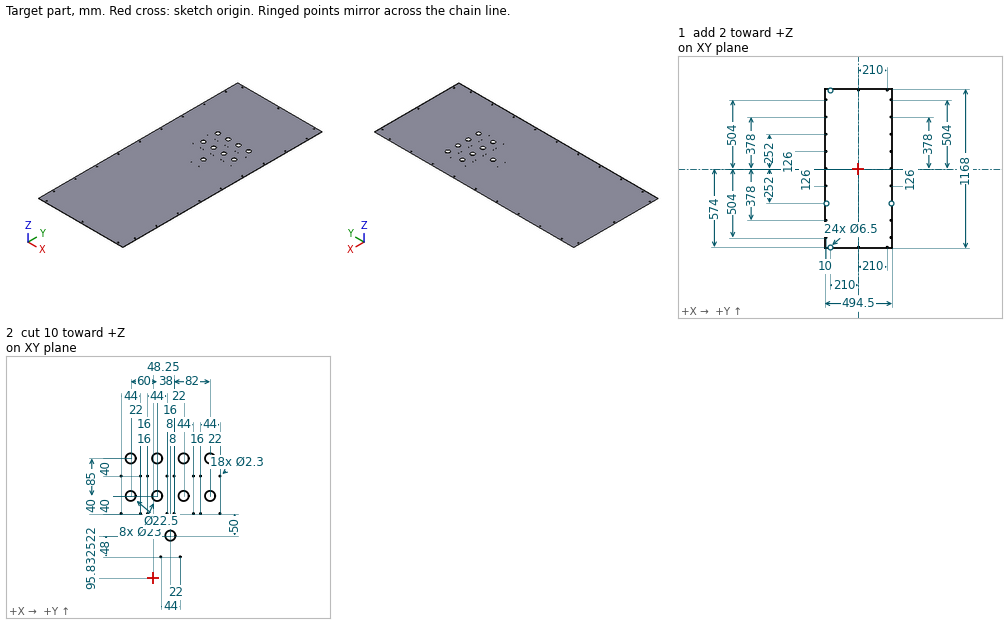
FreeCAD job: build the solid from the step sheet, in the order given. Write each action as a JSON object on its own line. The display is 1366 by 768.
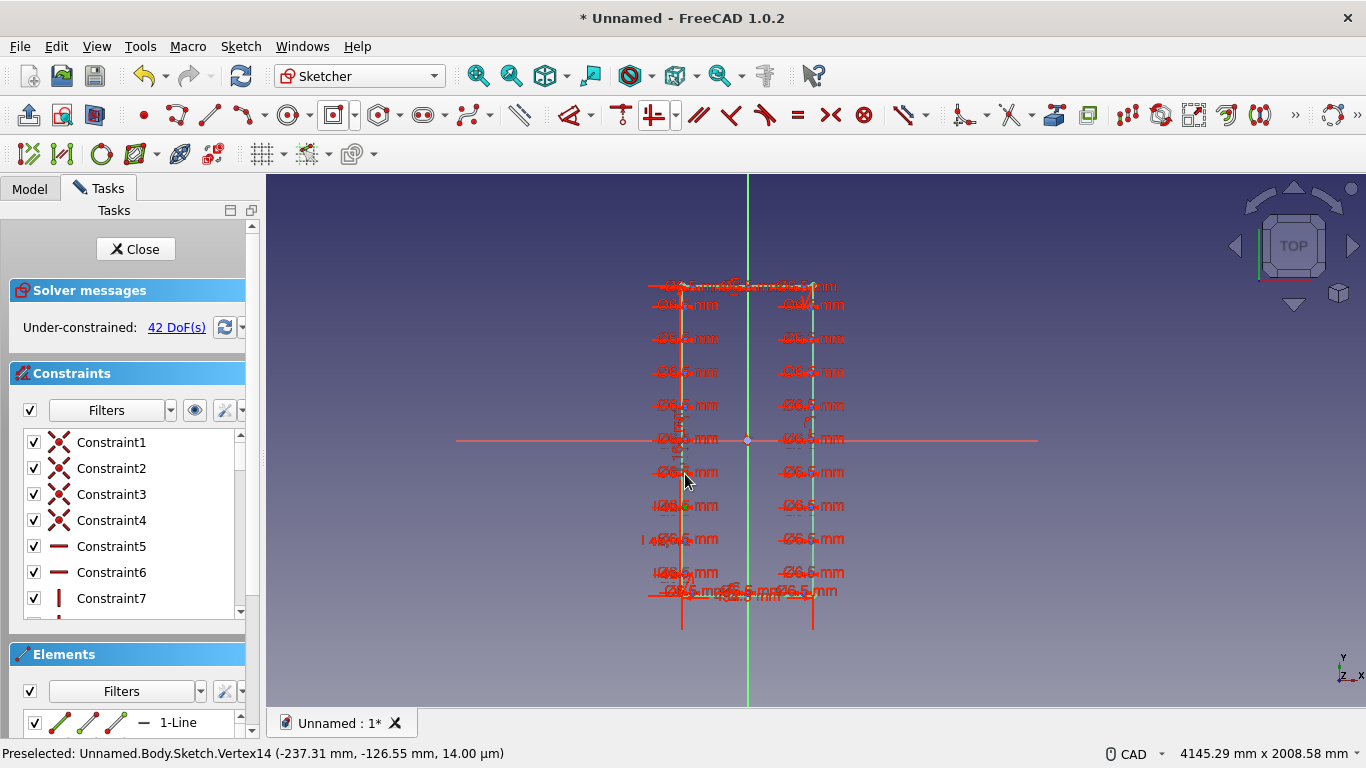
{"action": "key", "text": "v"}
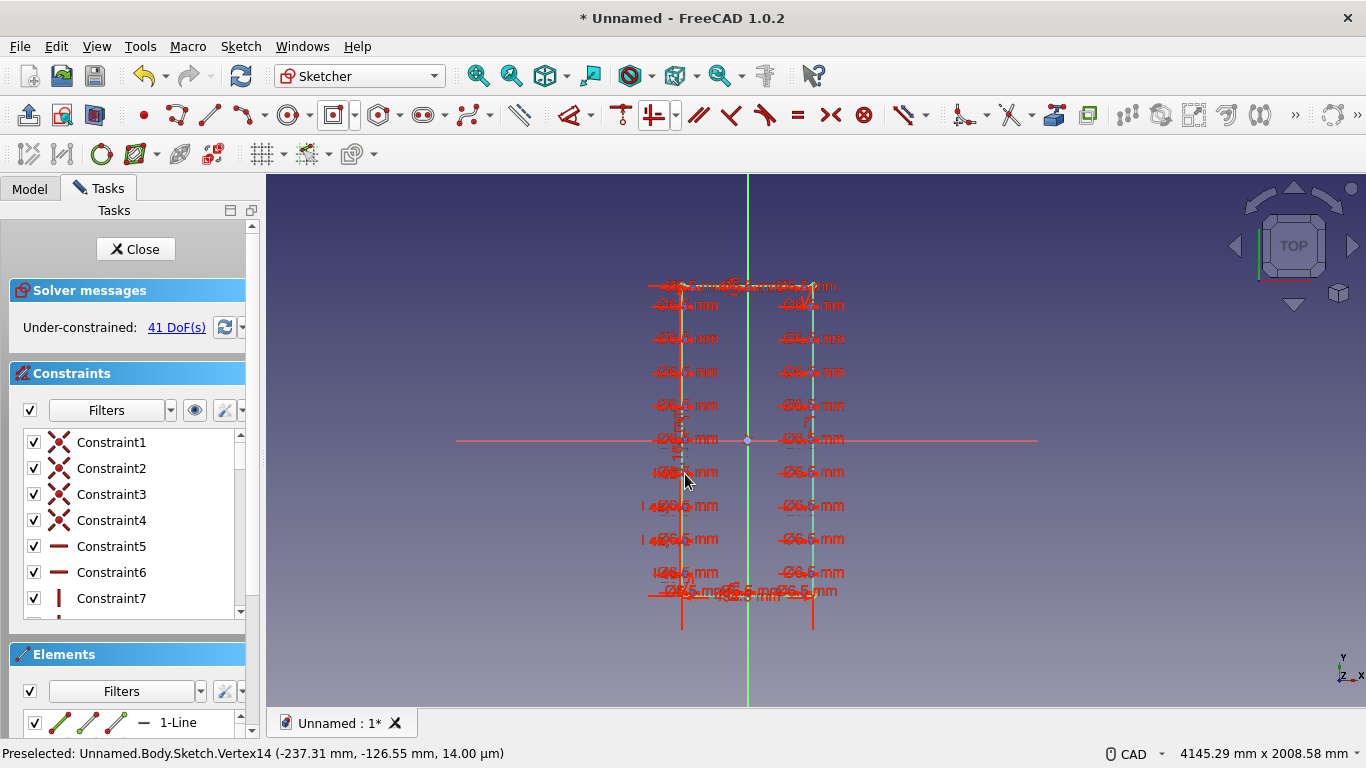
{"action": "left_click", "coordinate": [692, 593]}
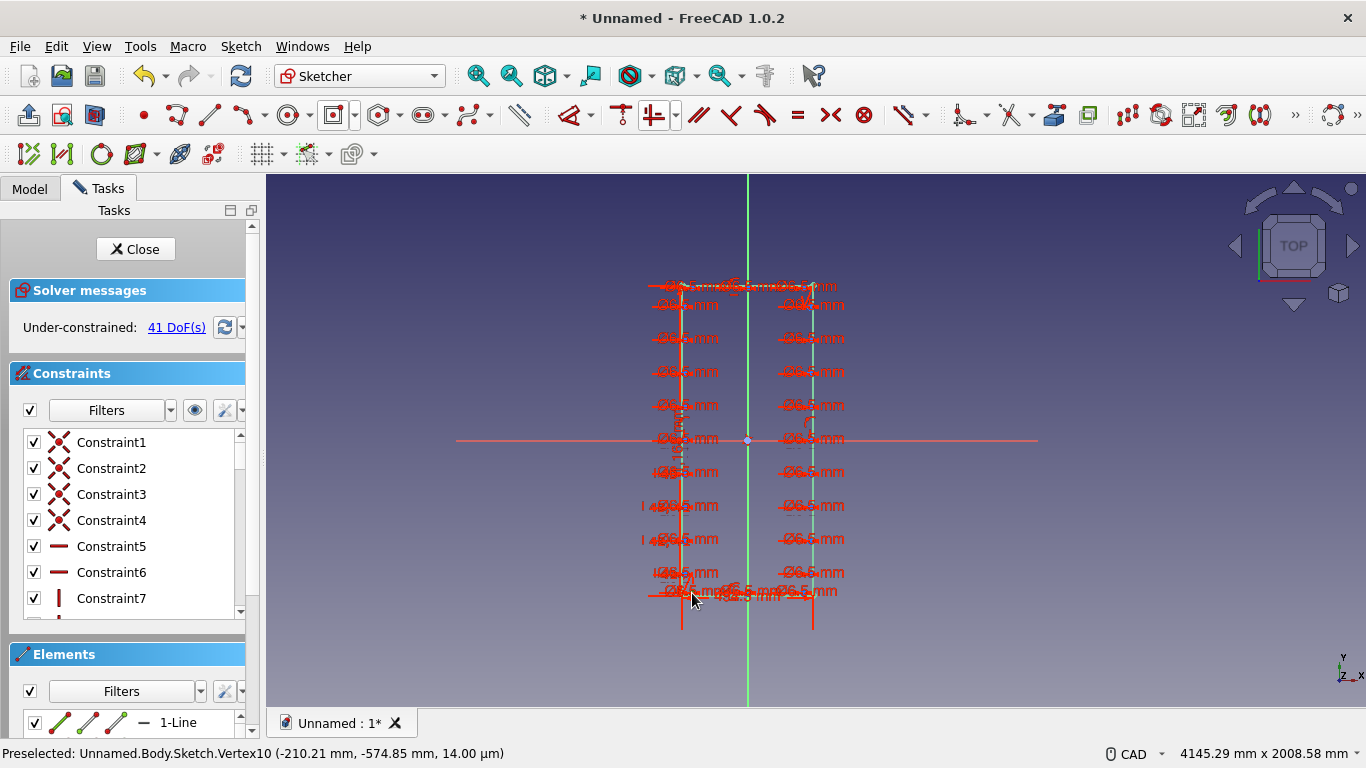
{"action": "left_click", "coordinate": [748, 593]}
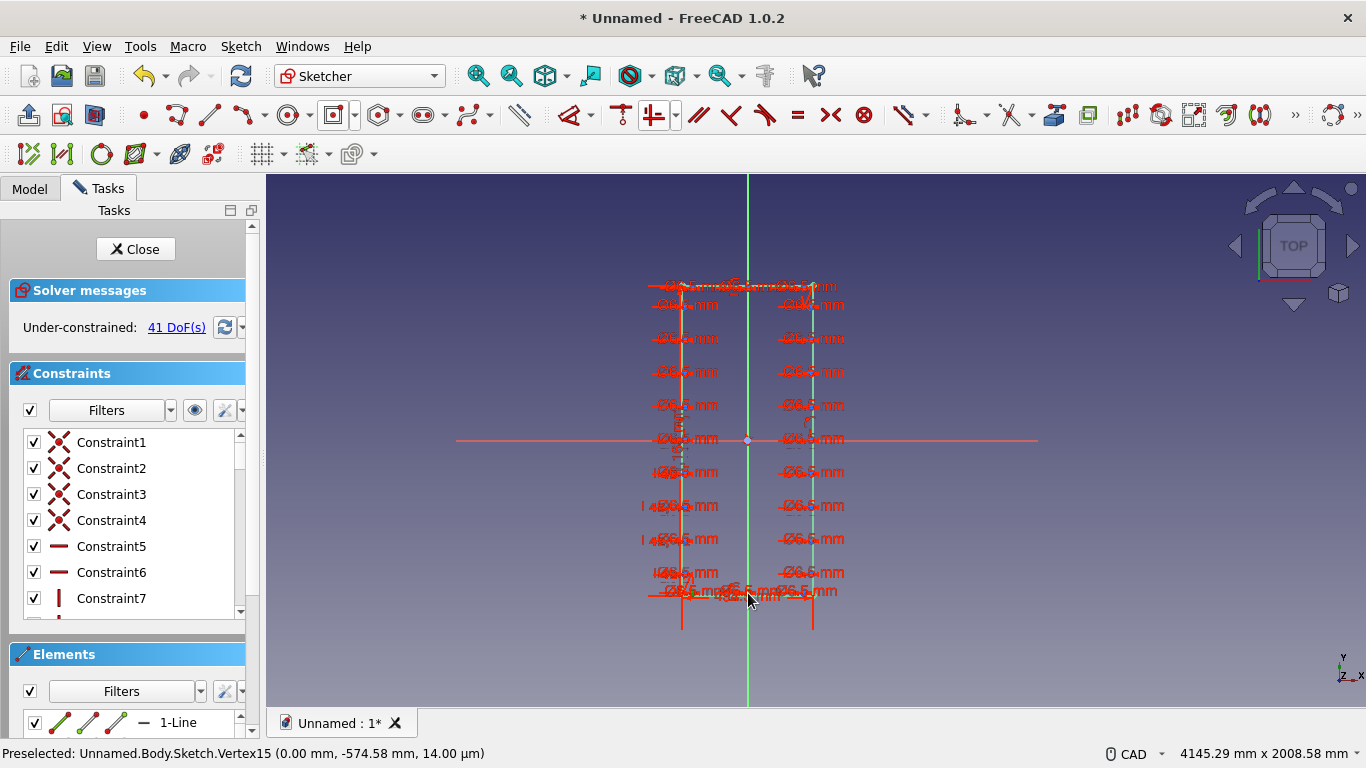
{"action": "left_click", "coordinate": [676, 116]}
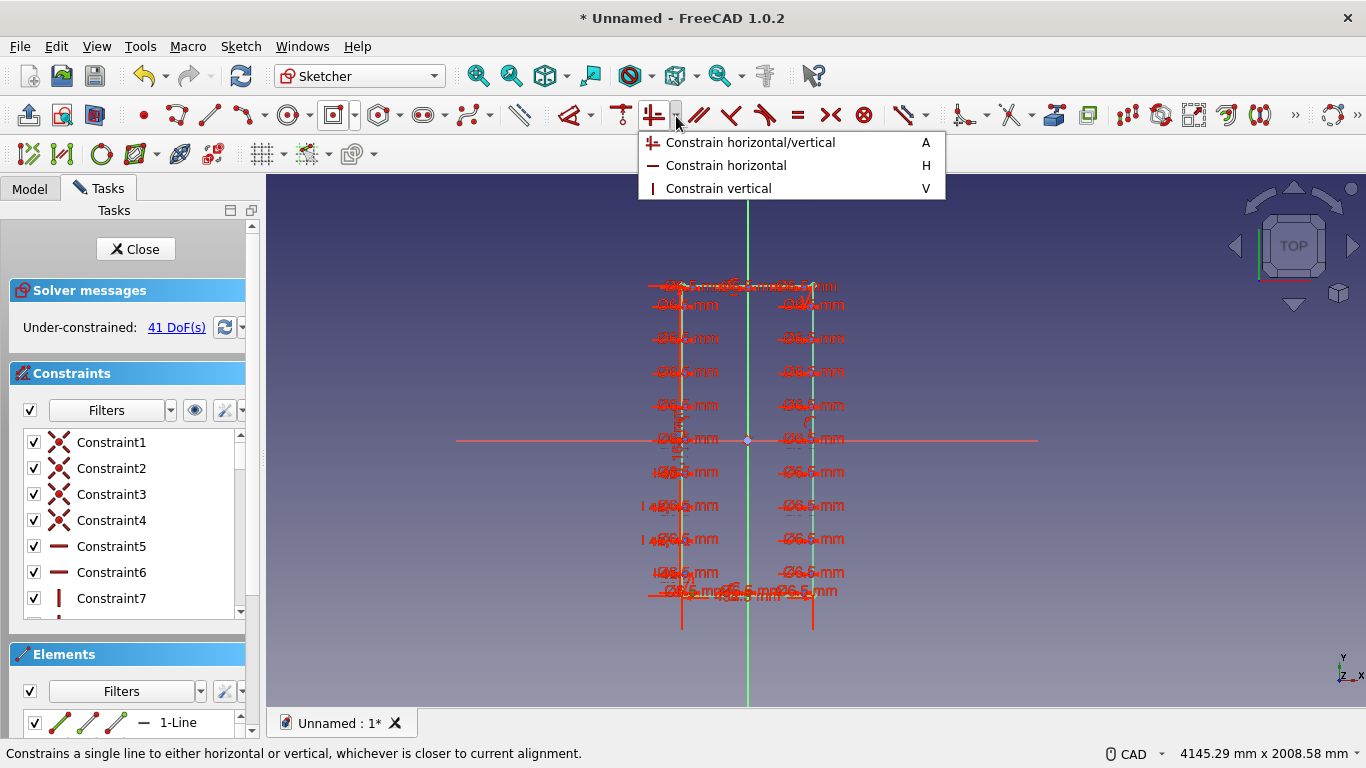
{"action": "left_click", "coordinate": [792, 166]}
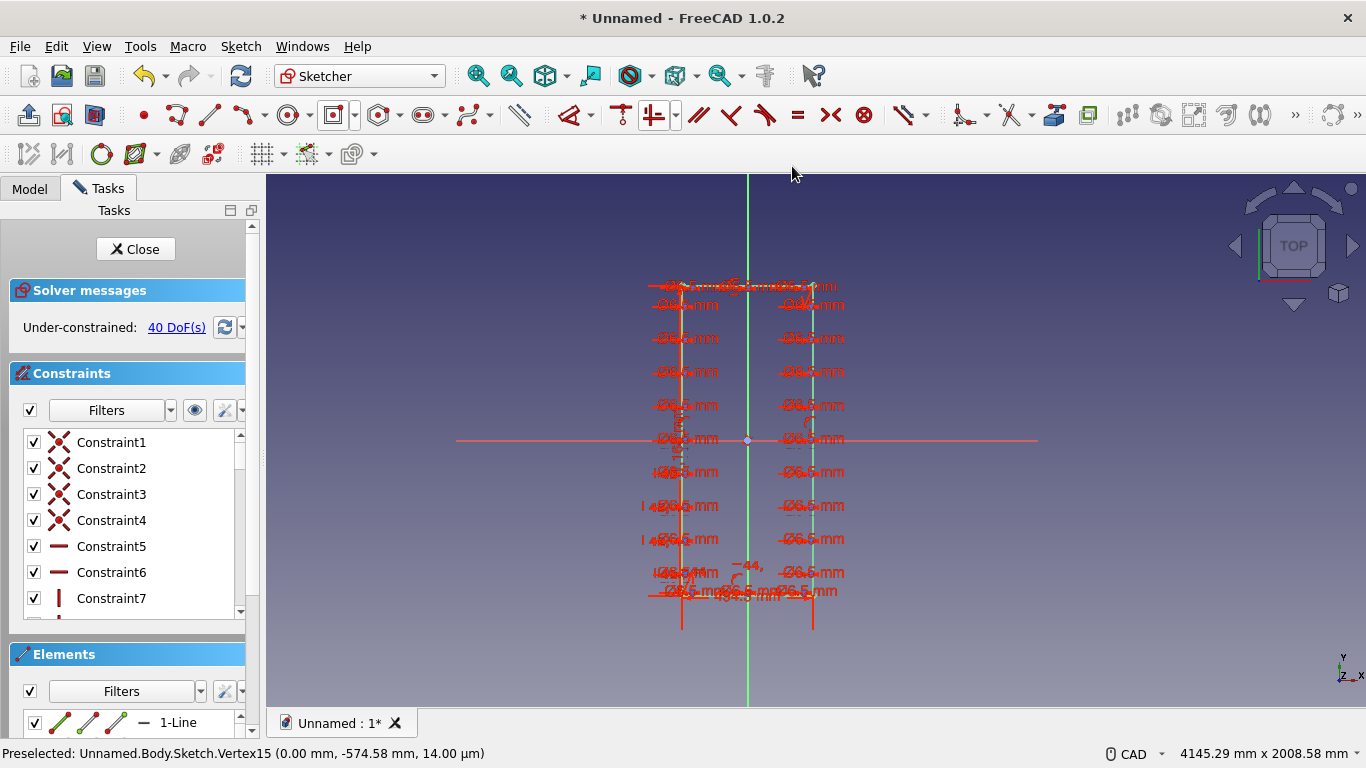
{"action": "left_click", "coordinate": [748, 593]}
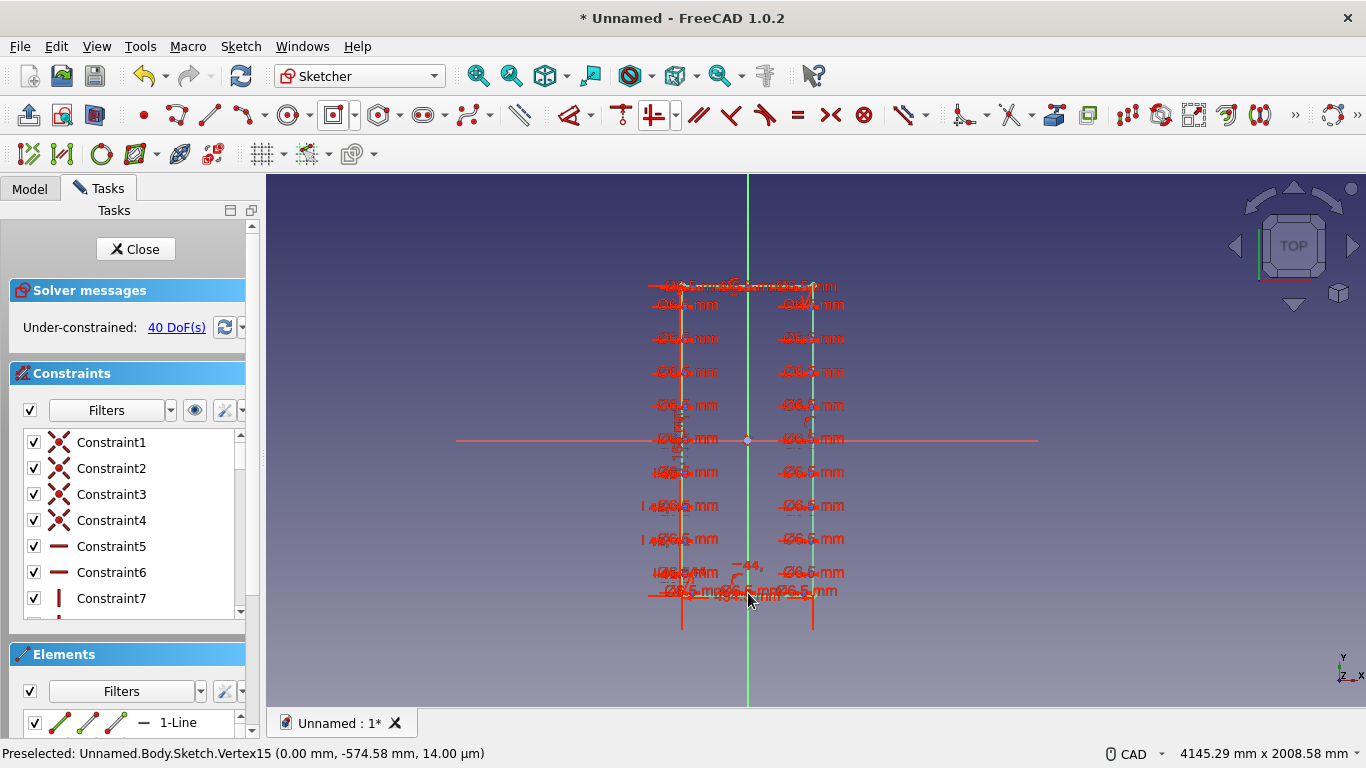
{"action": "left_click", "coordinate": [804, 593]}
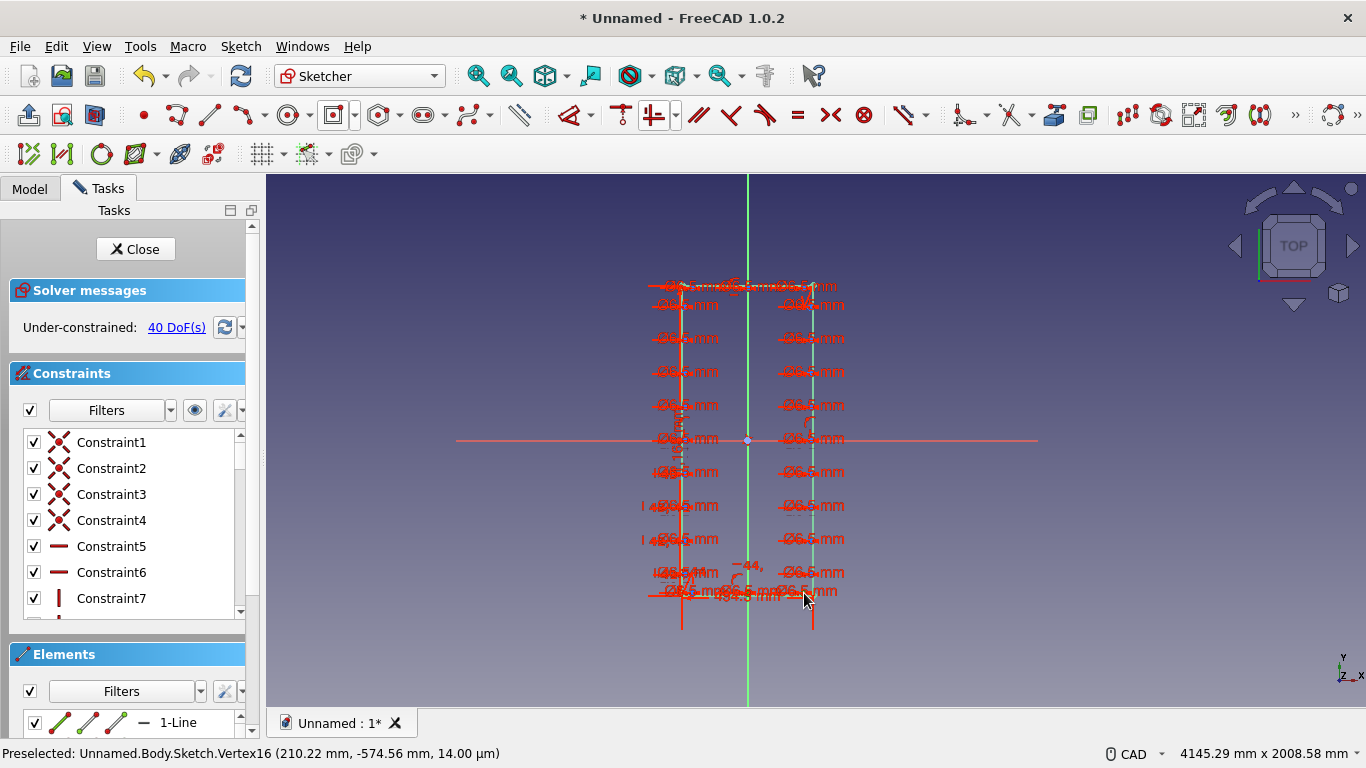
{"action": "left_click", "coordinate": [676, 116]}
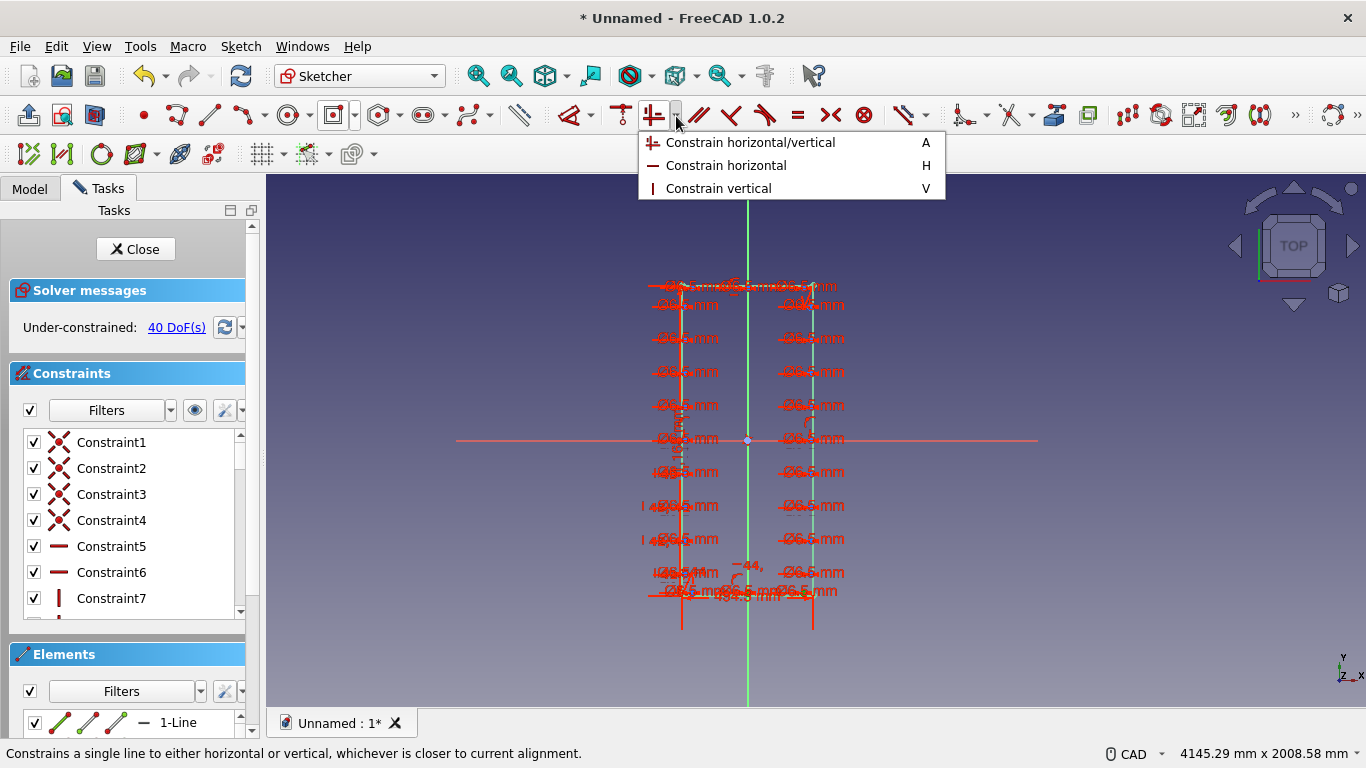
{"action": "left_click", "coordinate": [792, 166]}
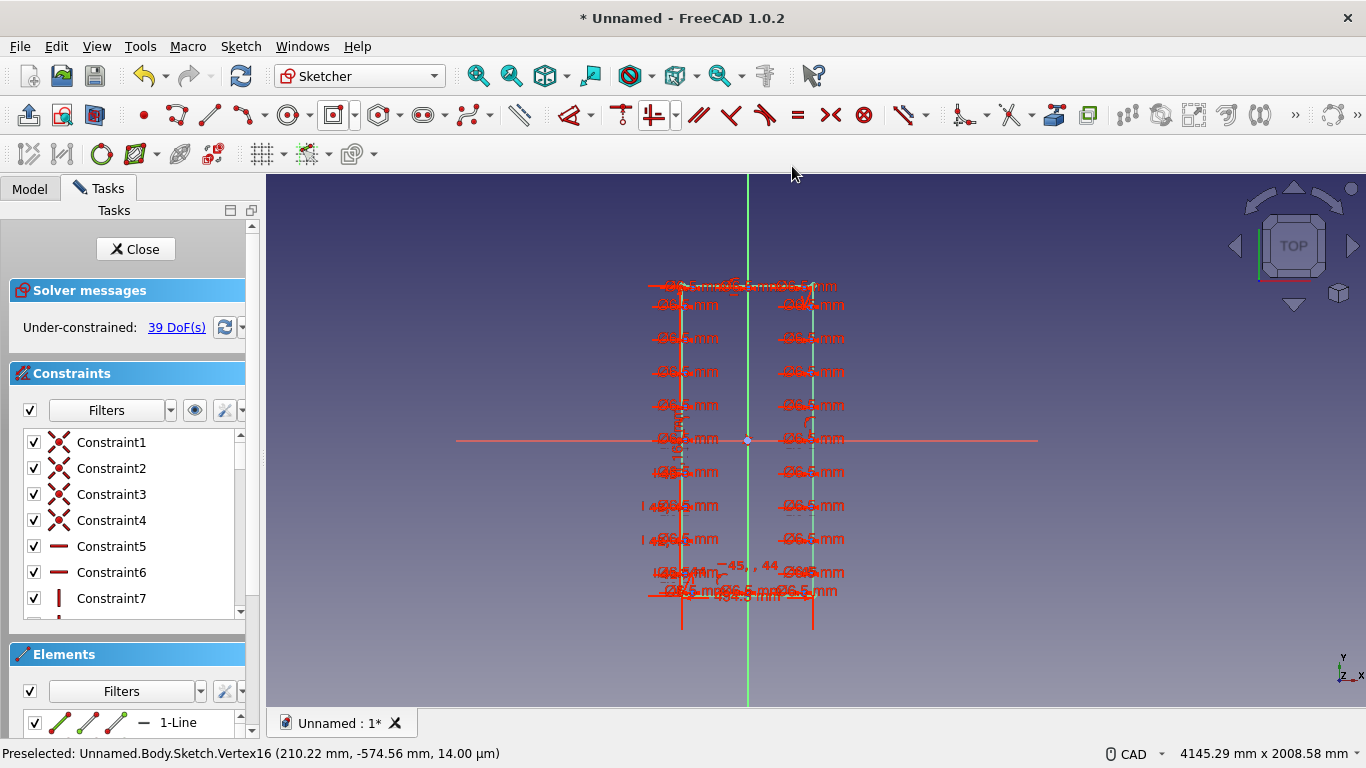
{"action": "left_click", "coordinate": [685, 575]}